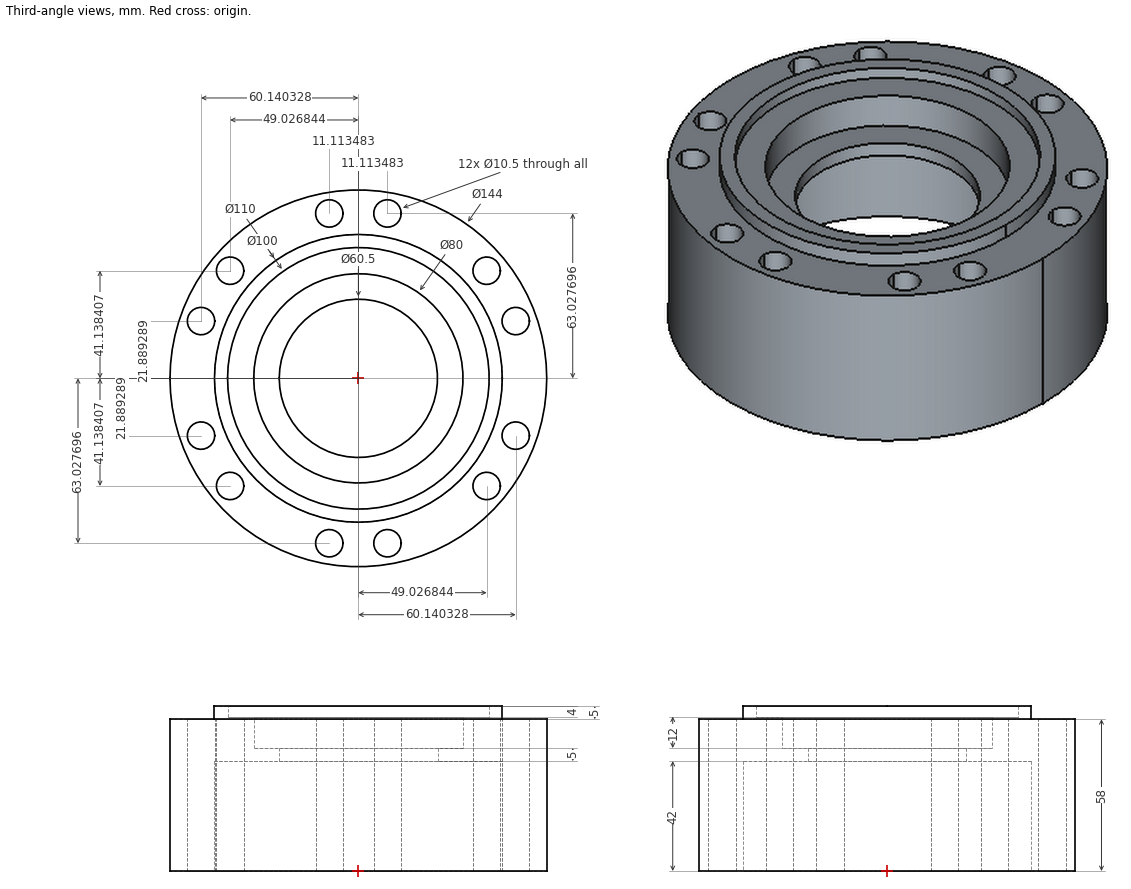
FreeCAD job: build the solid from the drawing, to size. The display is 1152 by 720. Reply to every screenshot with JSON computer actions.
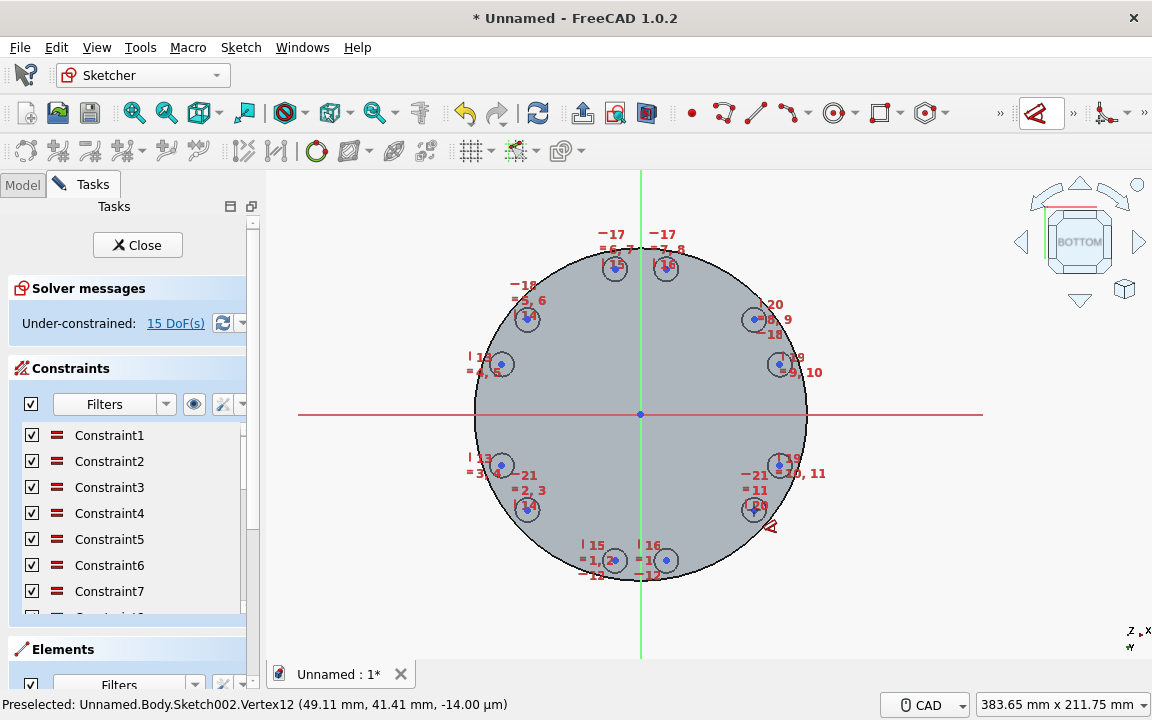
{"action": "scroll", "coordinate": [675, 552], "scroll_direction": "up", "scroll_amount": 3}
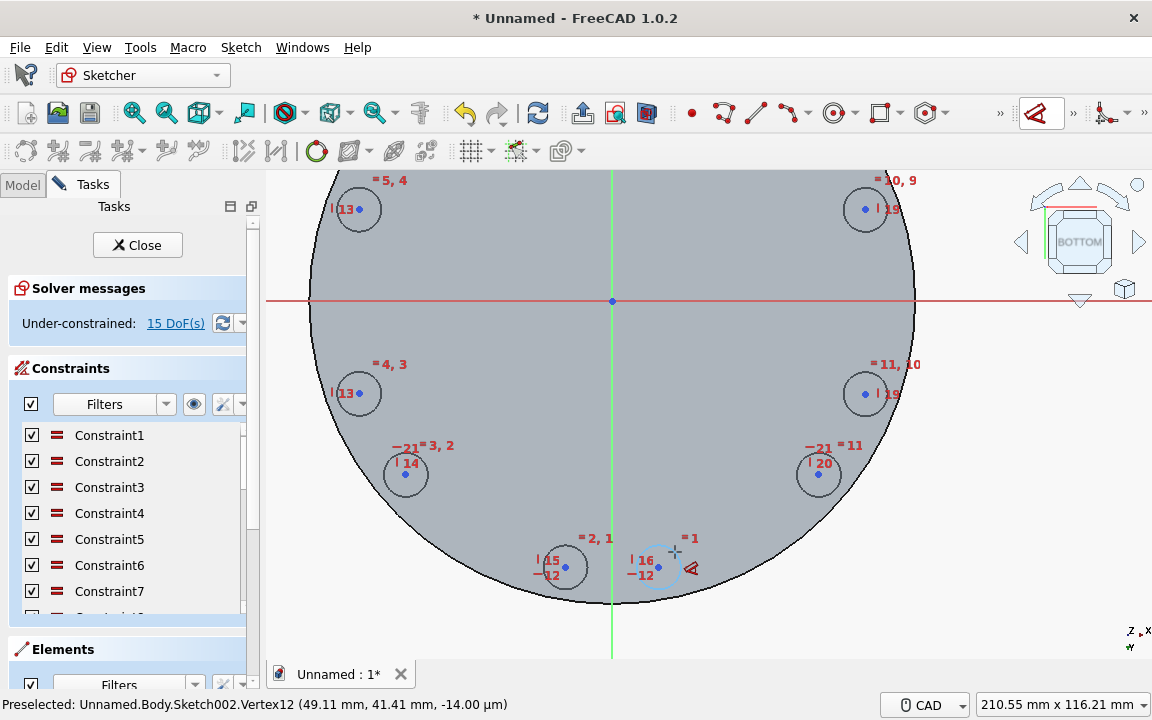
{"action": "left_click", "coordinate": [674, 552]}
{"action": "left_click", "coordinate": [696, 529]}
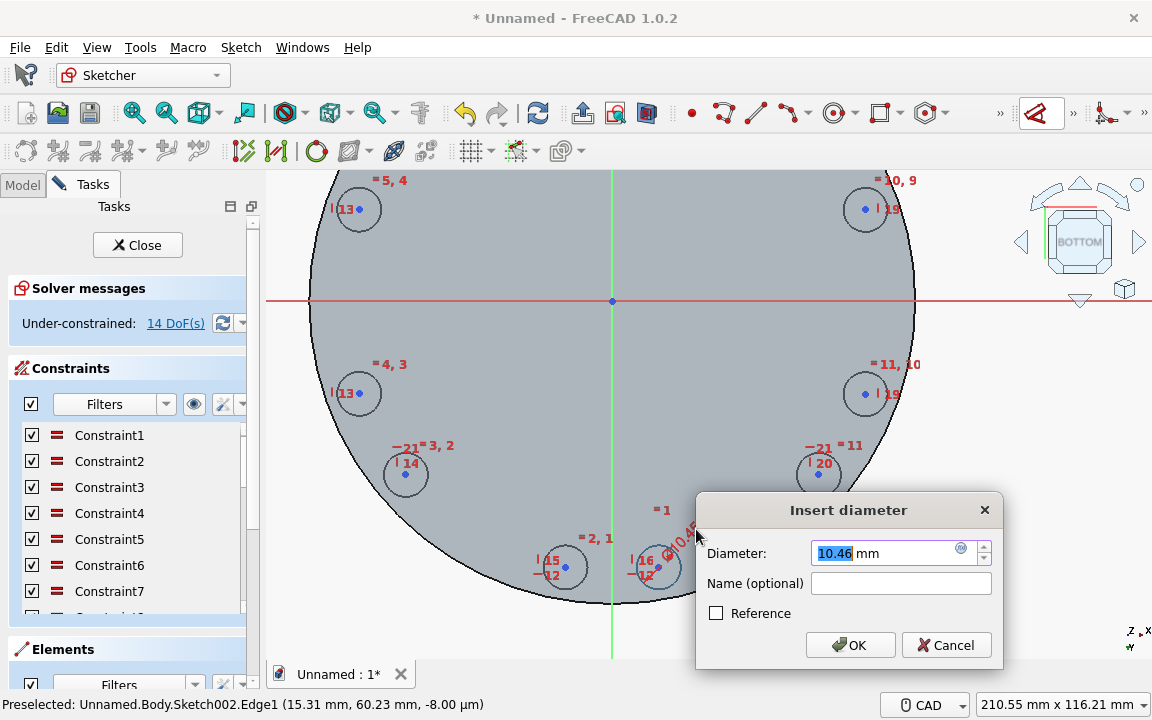
{"action": "type", "text": "10.5"}
{"action": "key", "text": "Return"}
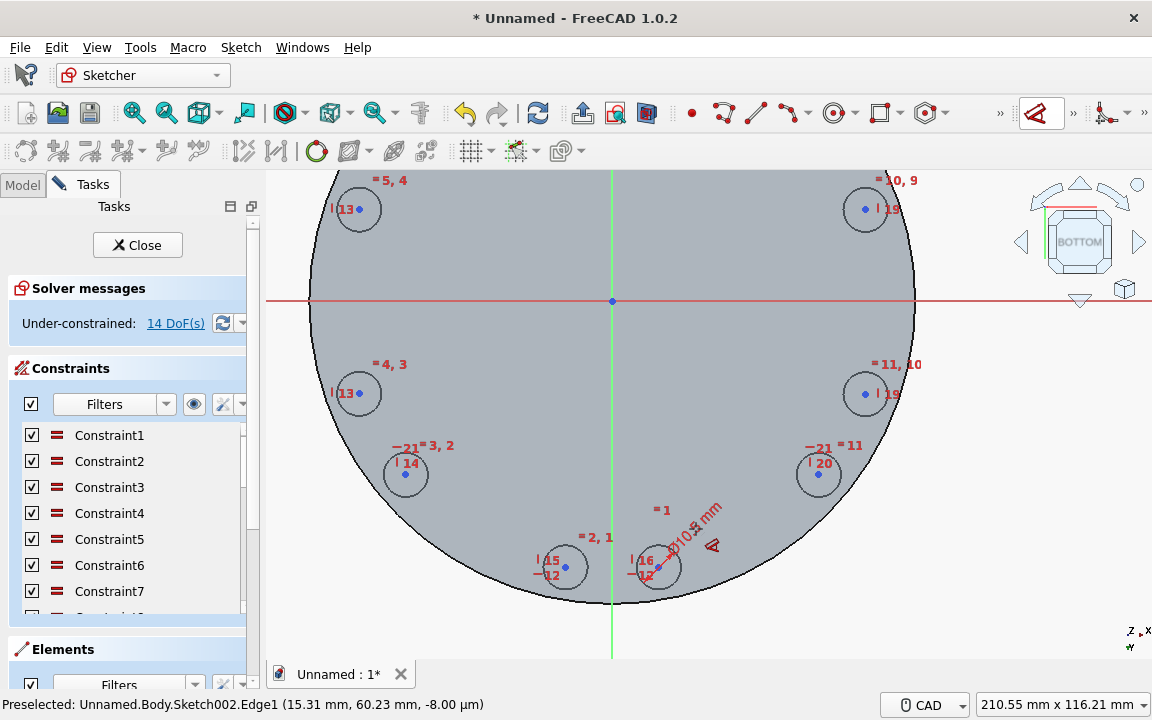
{"action": "left_click", "coordinate": [659, 567]}
{"action": "left_click", "coordinate": [636, 601]}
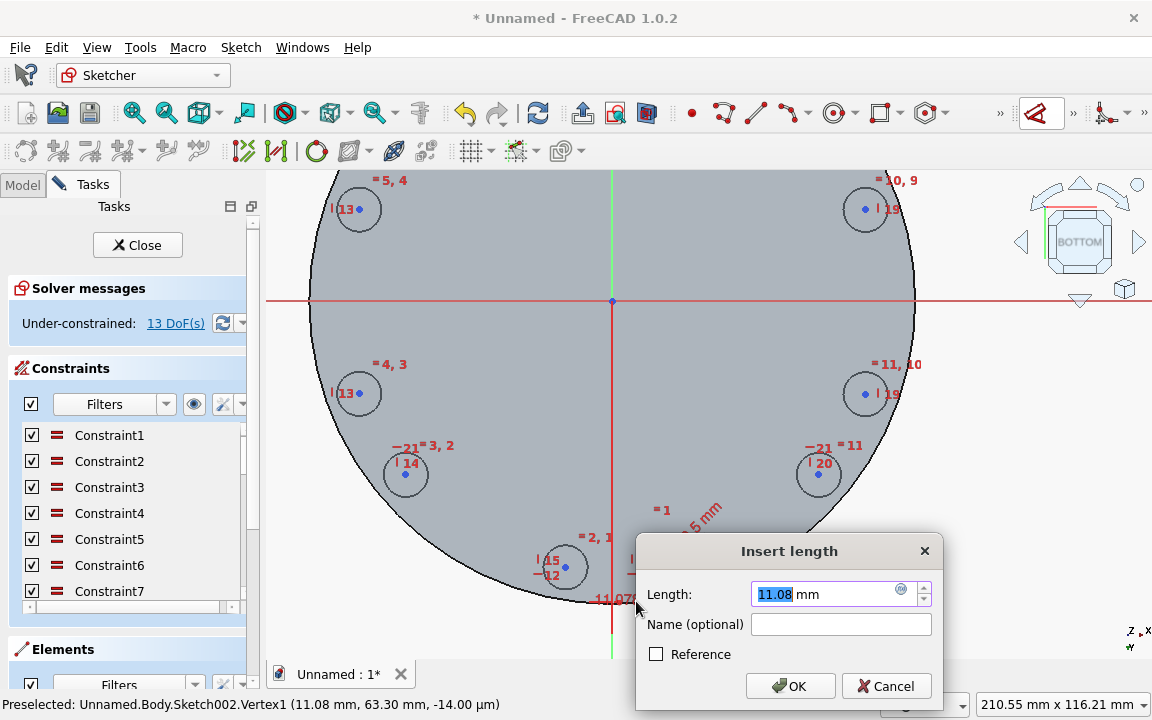
{"action": "type", "text": "11.113483"}
{"action": "key", "text": "Return"}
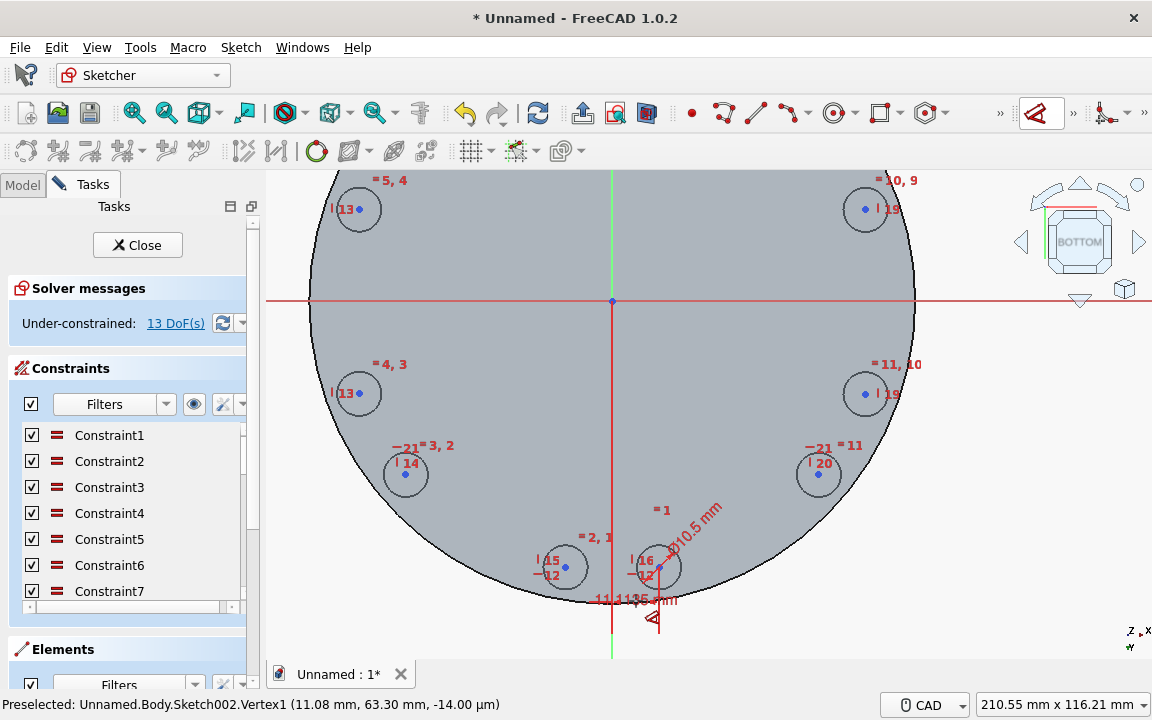
{"action": "left_click", "coordinate": [659, 567]}
{"action": "left_click", "coordinate": [693, 434]}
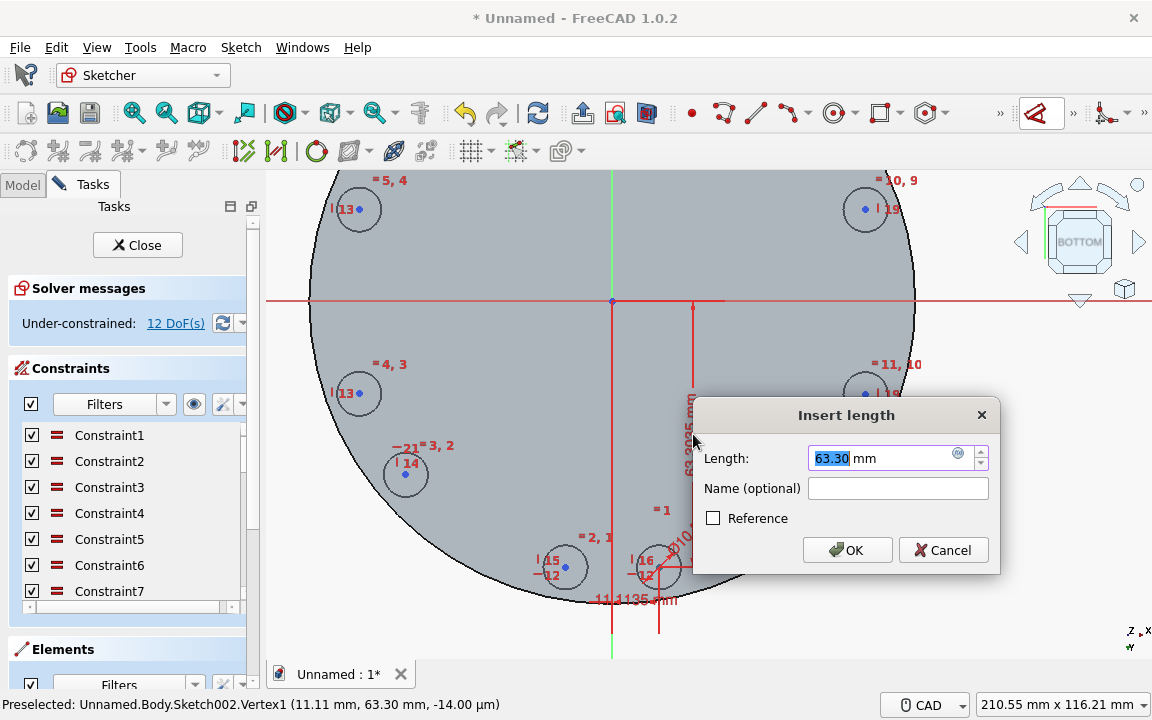
{"action": "type", "text": "63.027696"}
{"action": "key", "text": "Return"}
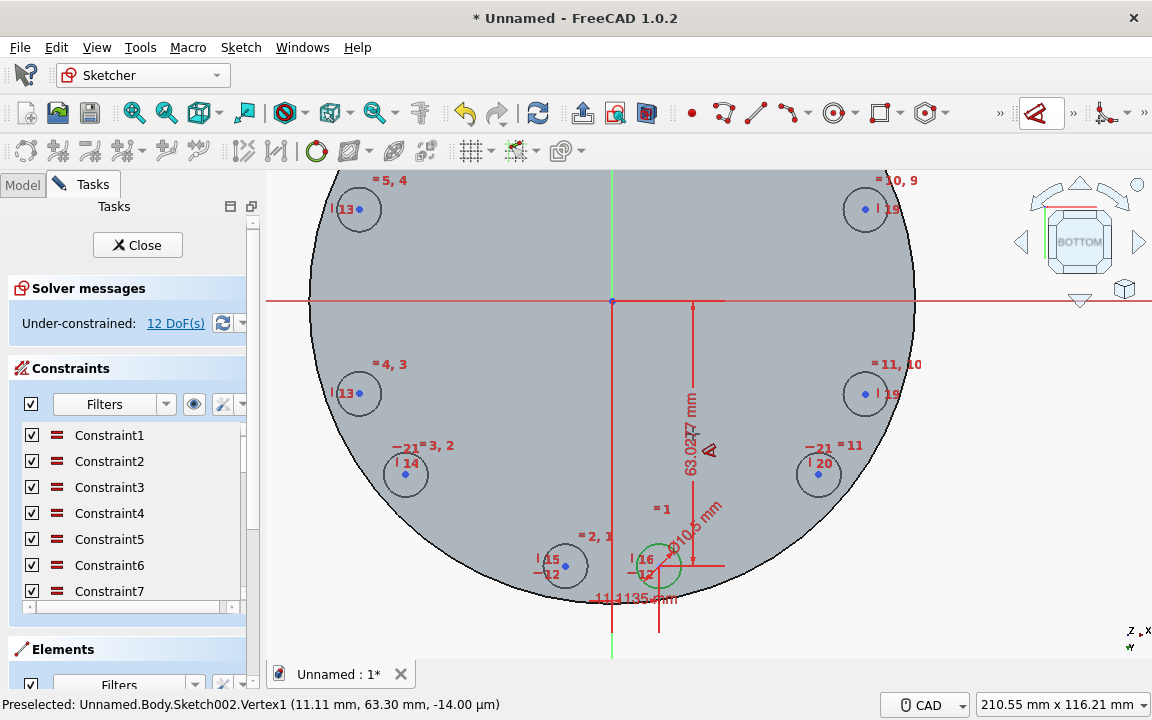
{"action": "left_click", "coordinate": [566, 566]}
{"action": "left_click", "coordinate": [589, 267]}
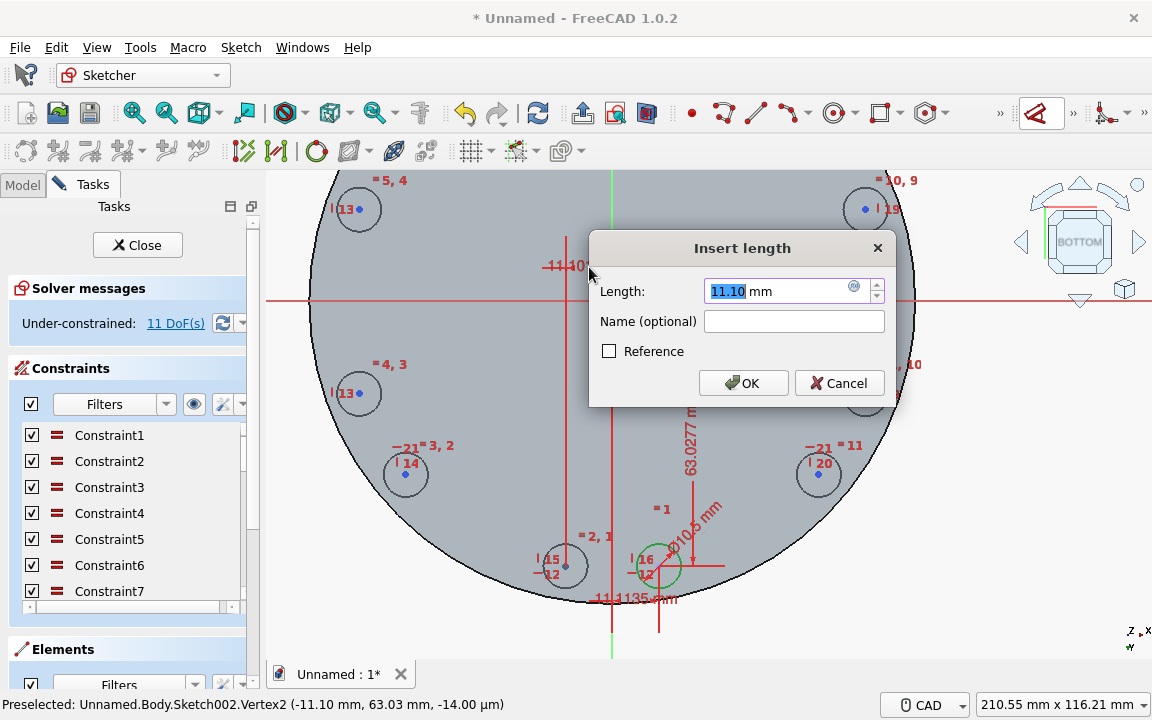
{"action": "type", "text": "11.113483"}
{"action": "key", "text": "Return"}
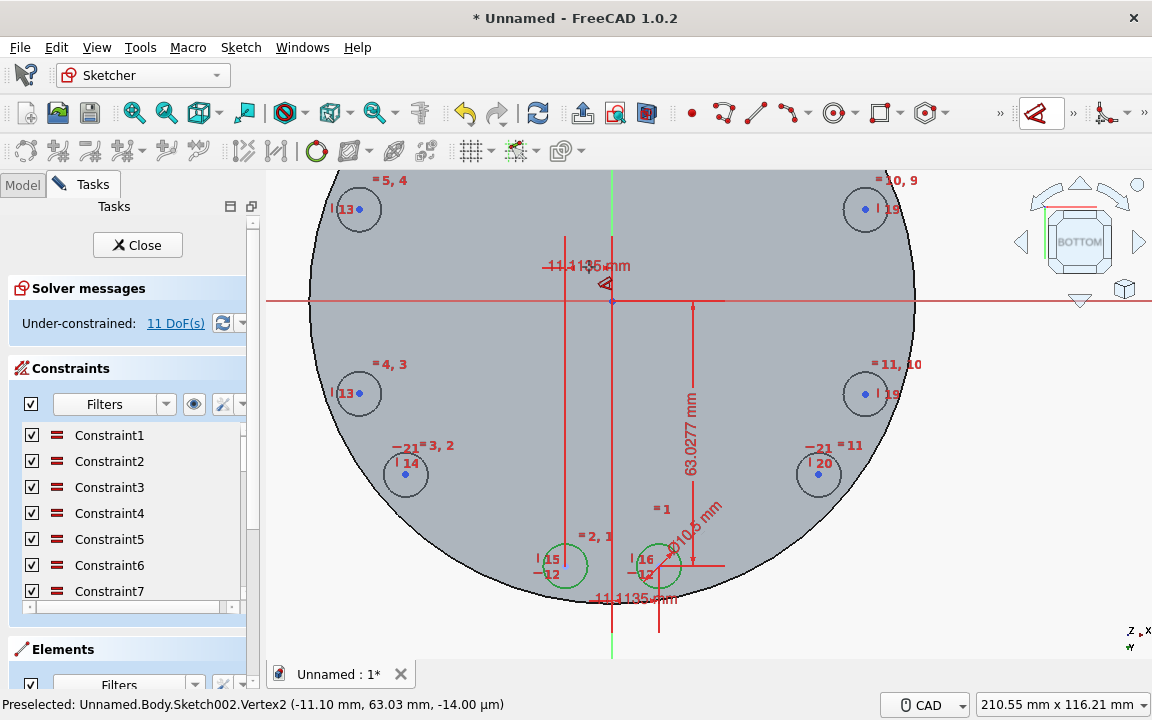
{"action": "left_click", "coordinate": [406, 475]}
{"action": "left_click", "coordinate": [509, 509]}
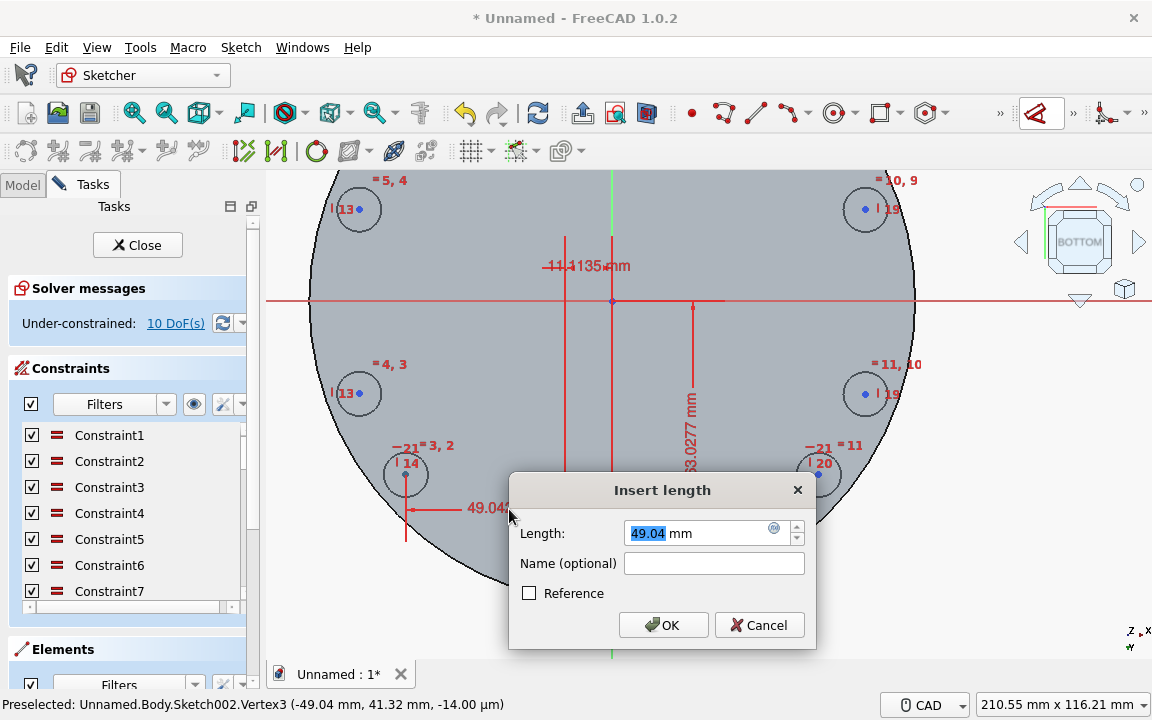
{"action": "type", "text": "49.026844"}
{"action": "key", "text": "Return"}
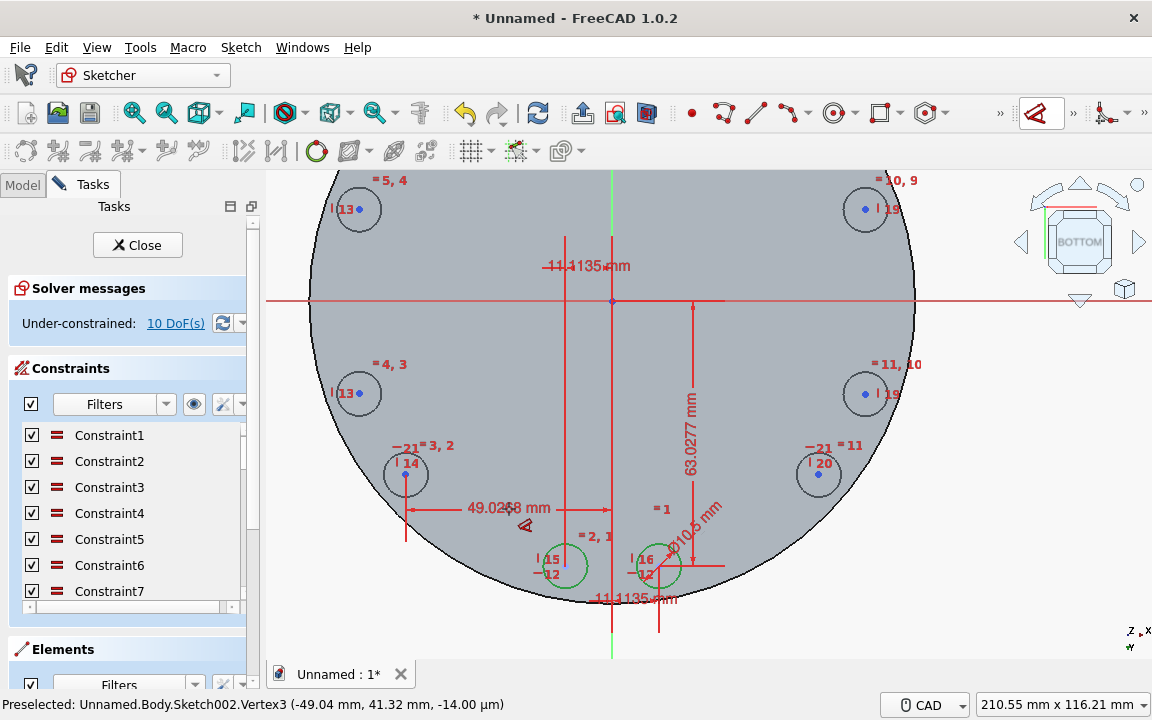
{"action": "left_click", "coordinate": [406, 475]}
{"action": "left_click", "coordinate": [372, 348]}